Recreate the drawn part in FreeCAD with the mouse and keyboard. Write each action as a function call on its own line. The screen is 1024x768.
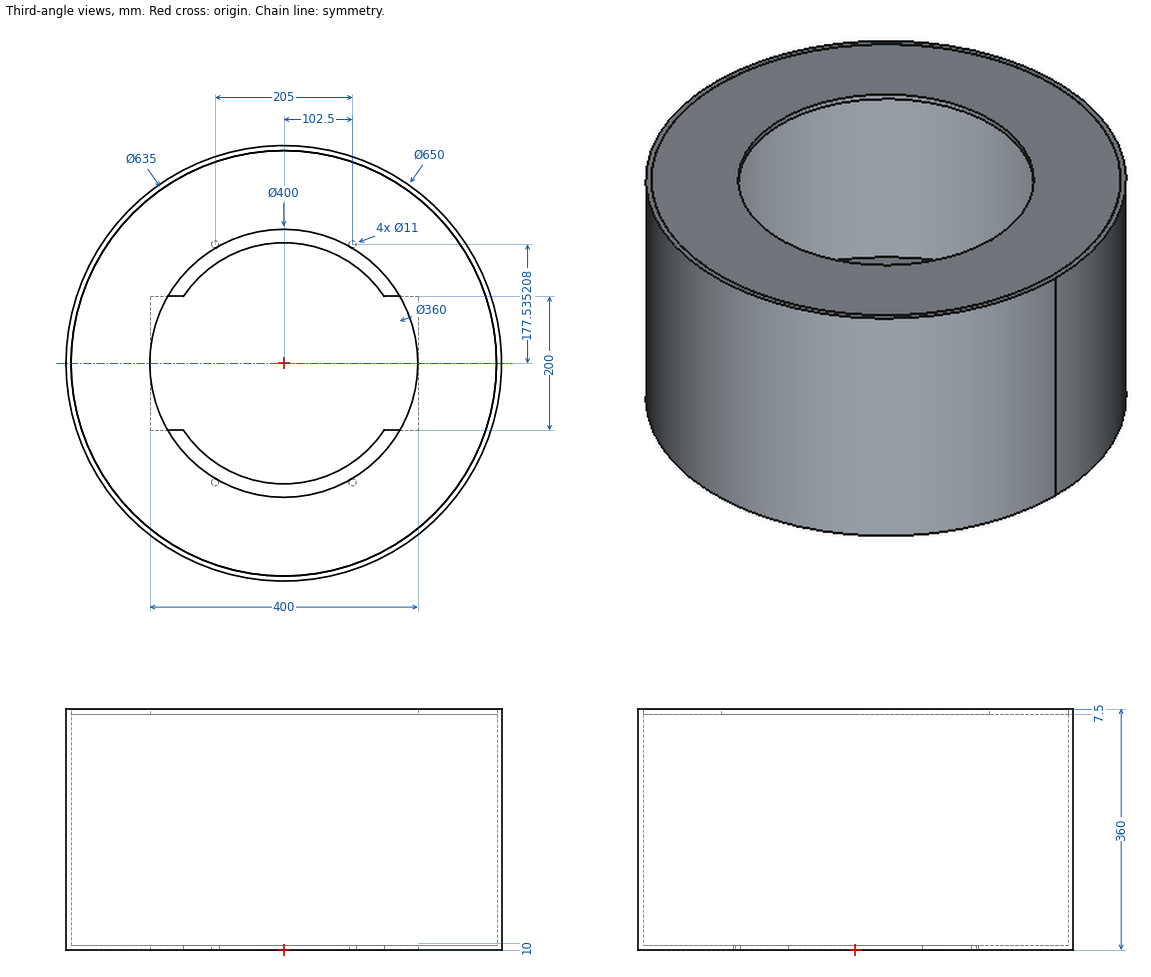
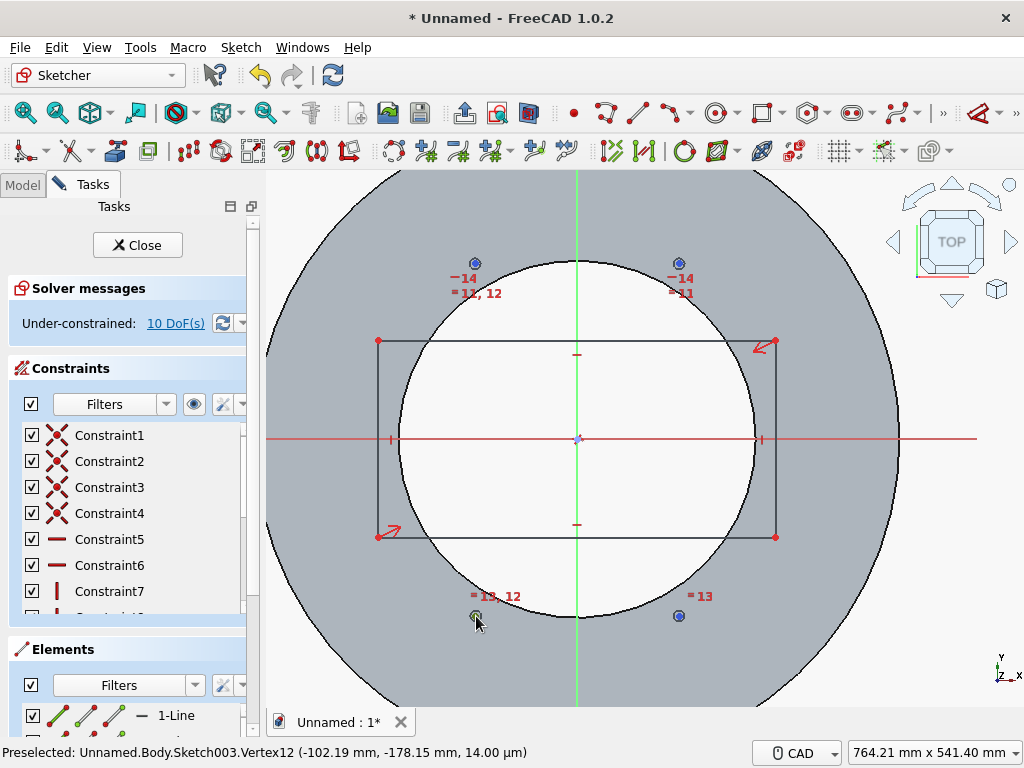
click(679, 616)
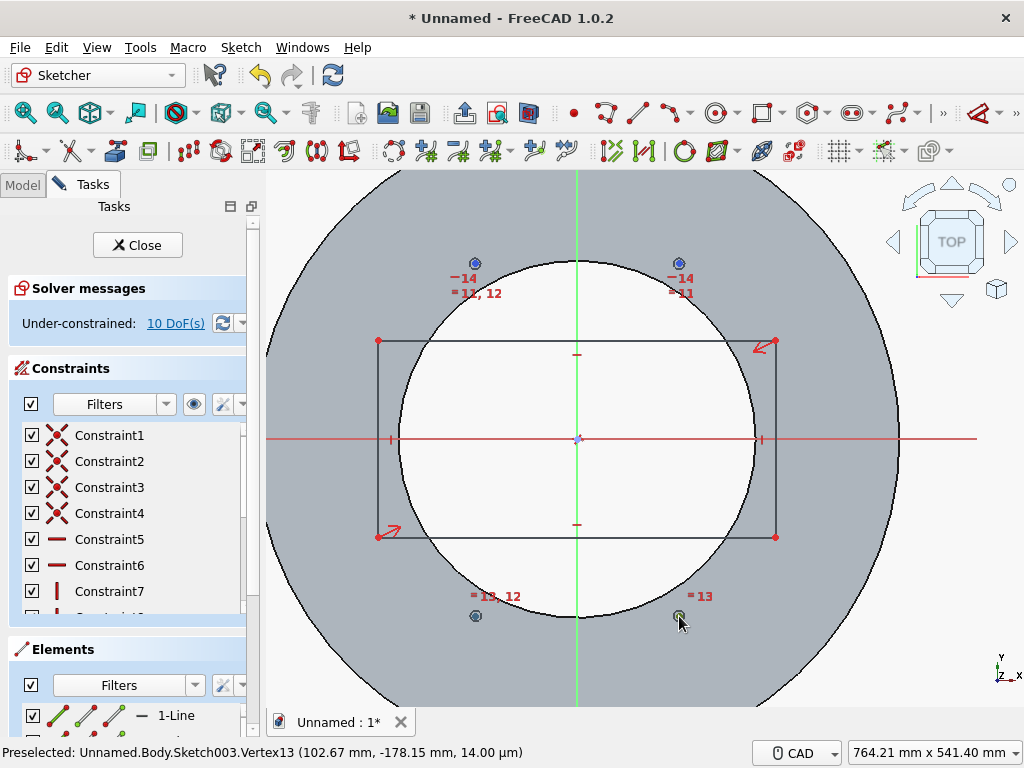
key(h)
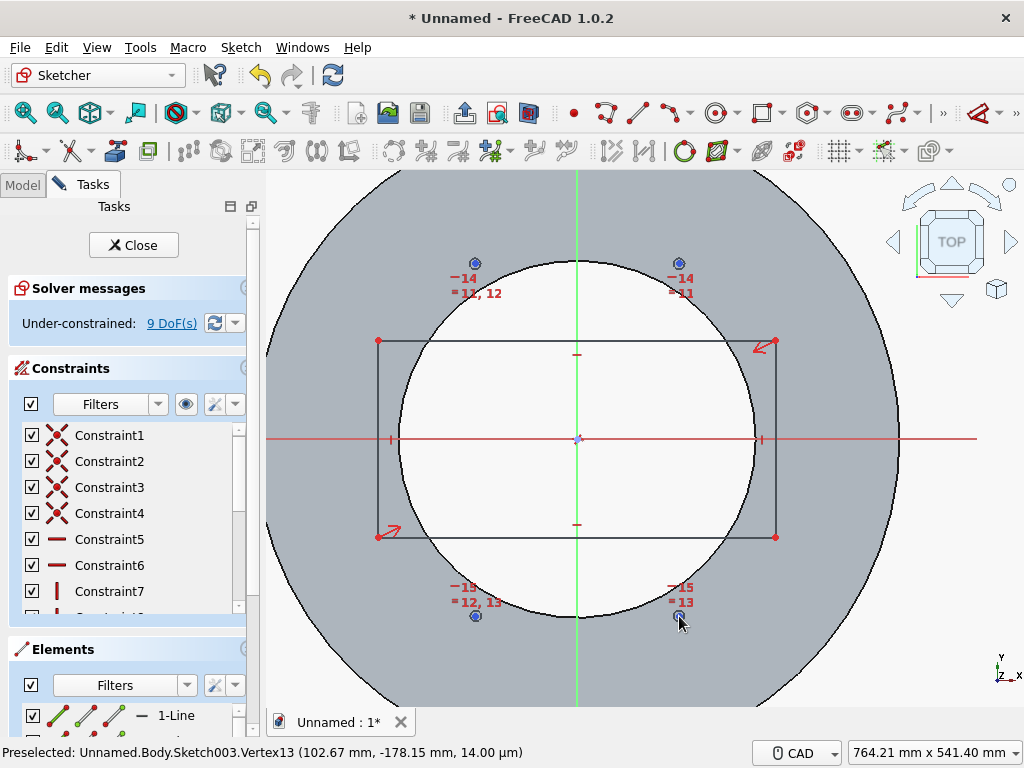
click(475, 264)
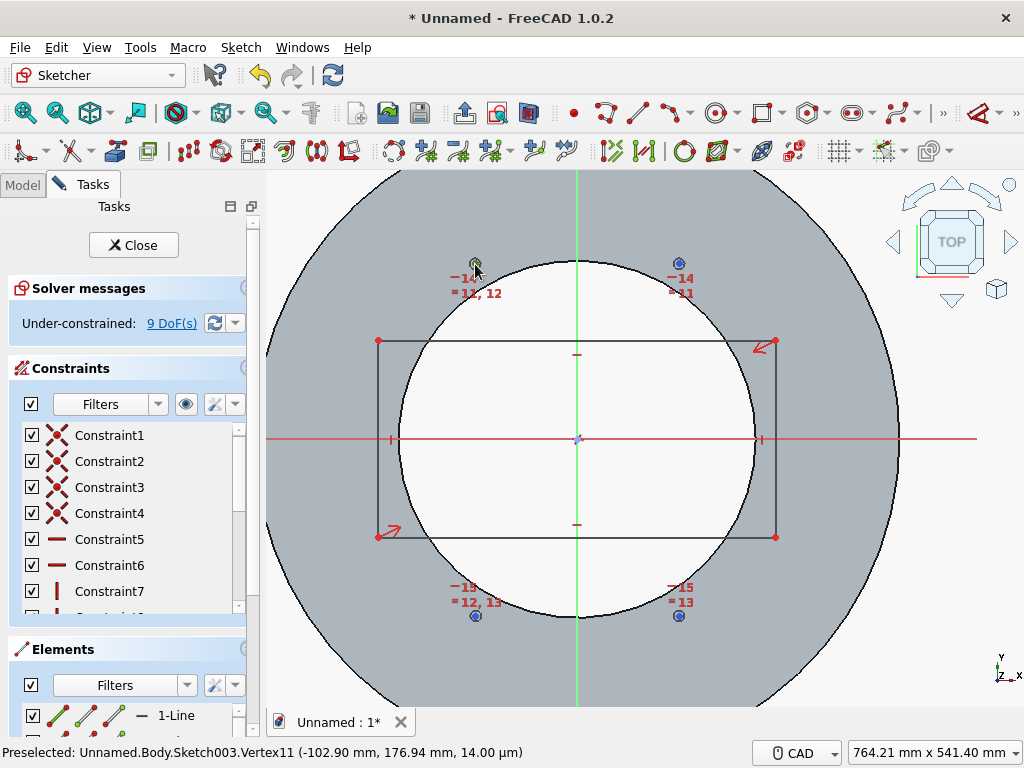
click(476, 616)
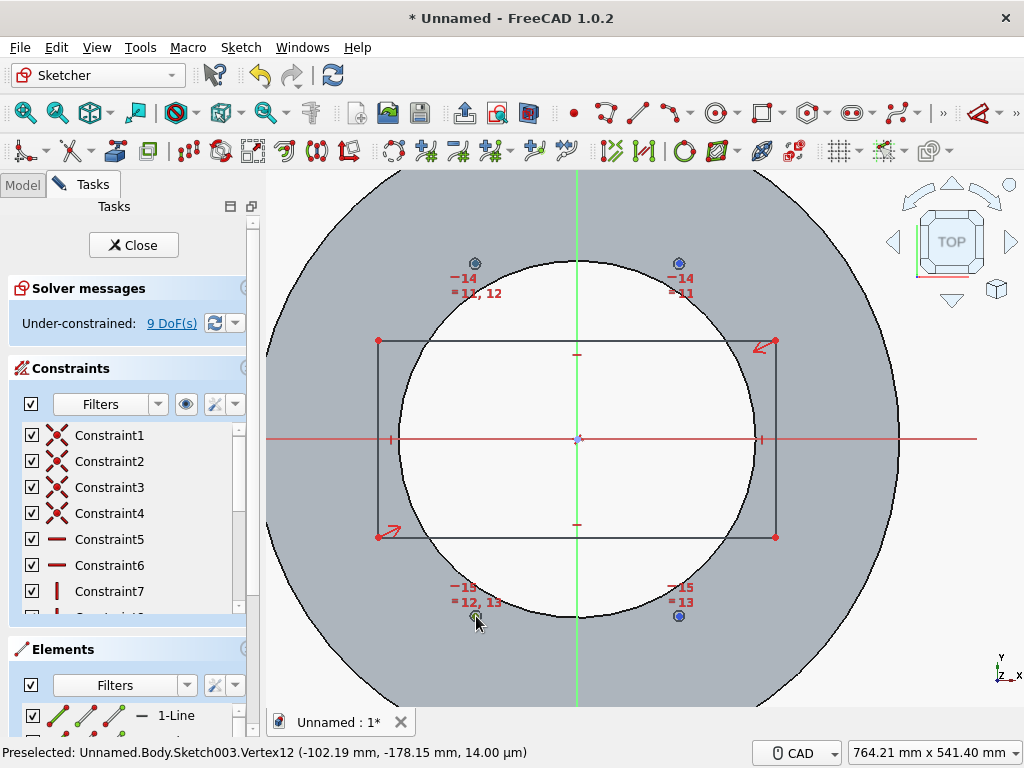
click(334, 439)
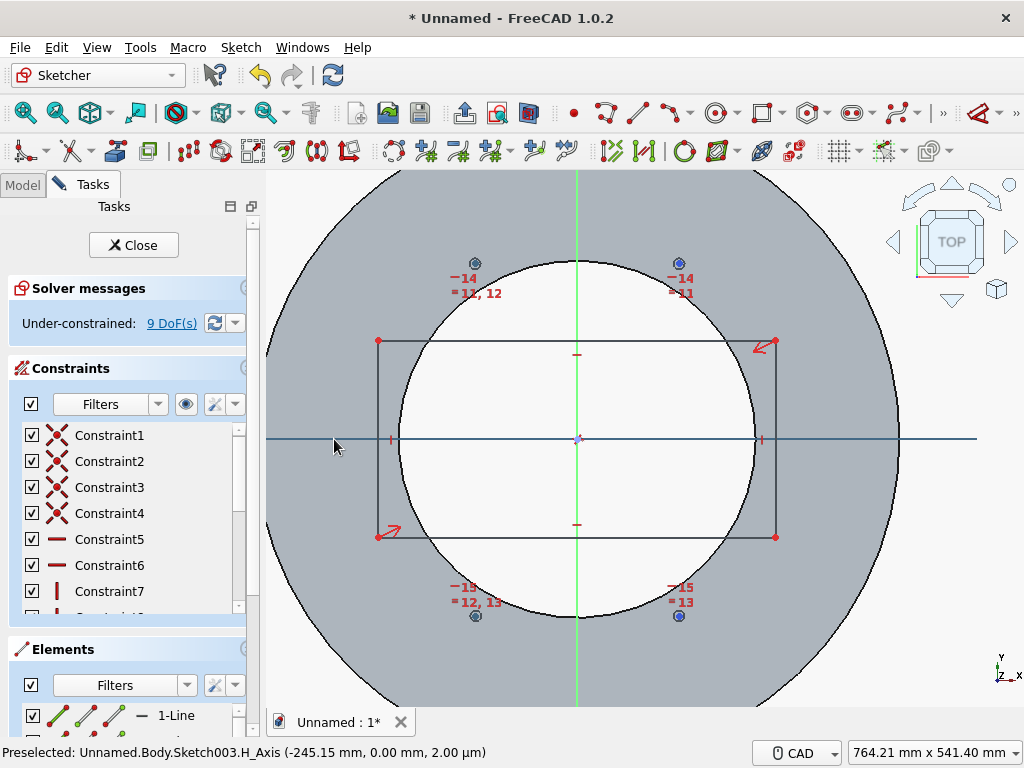
key(s)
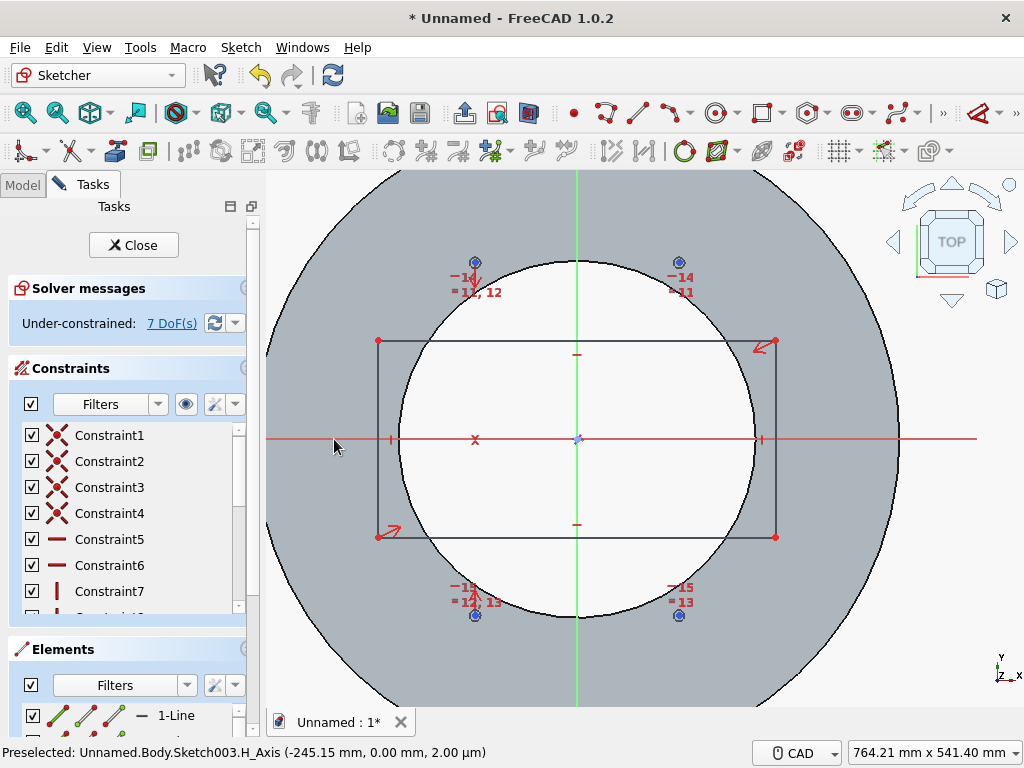
click(978, 114)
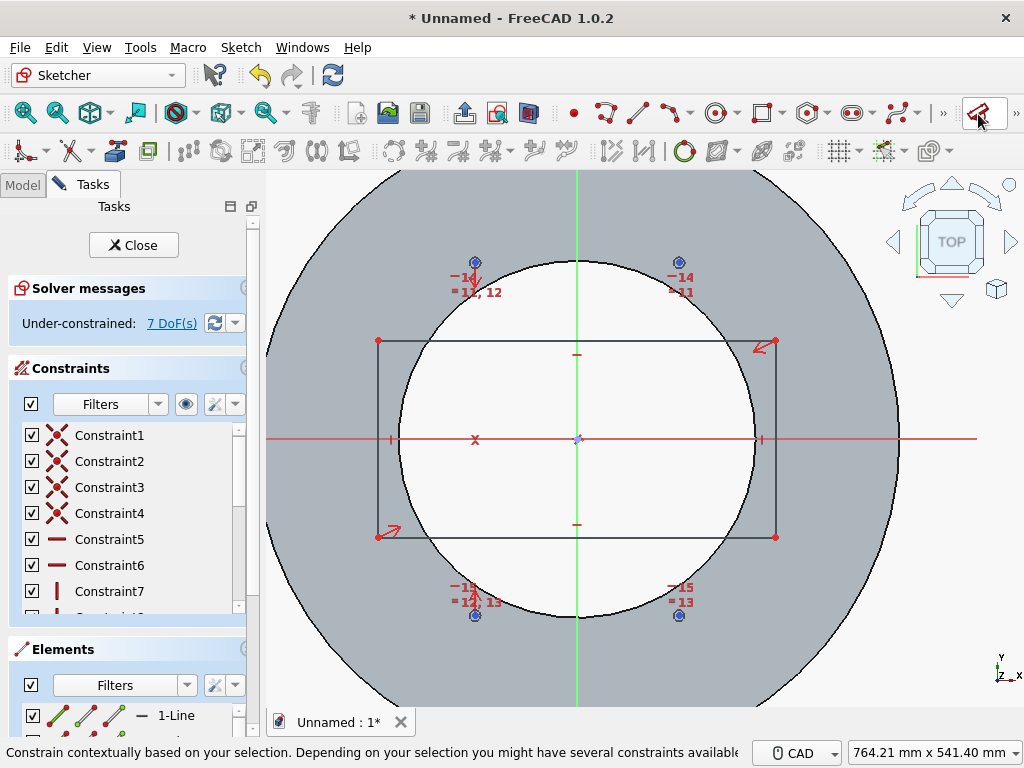
scroll(679, 257, up, 7)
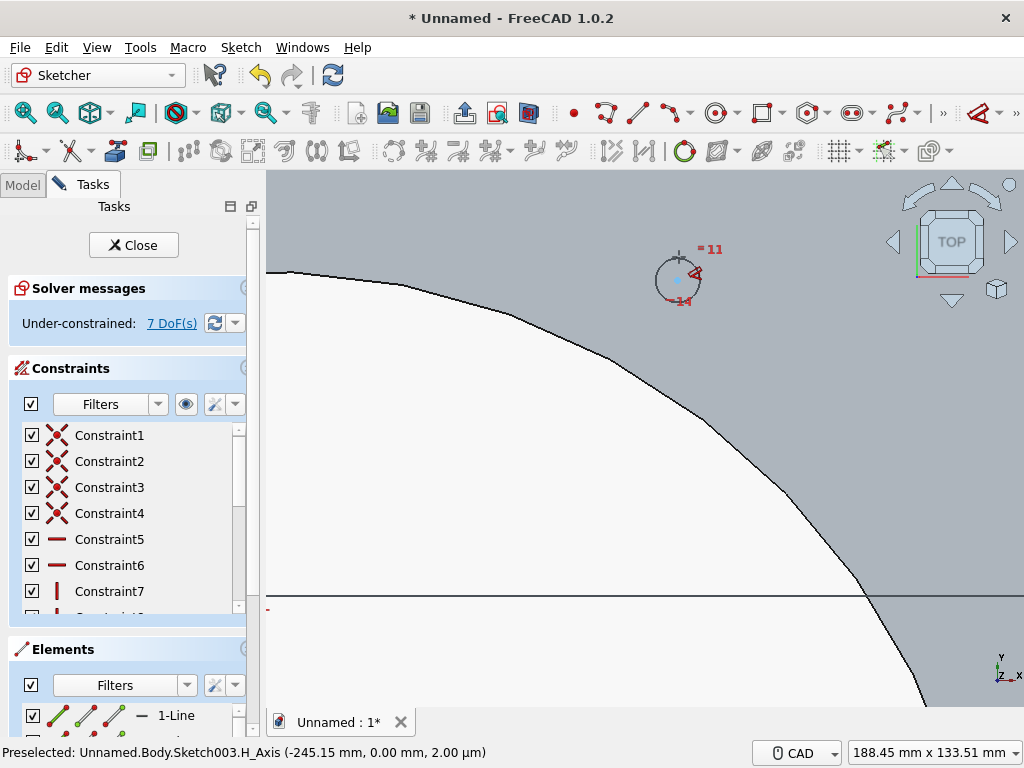
click(678, 258)
click(678, 226)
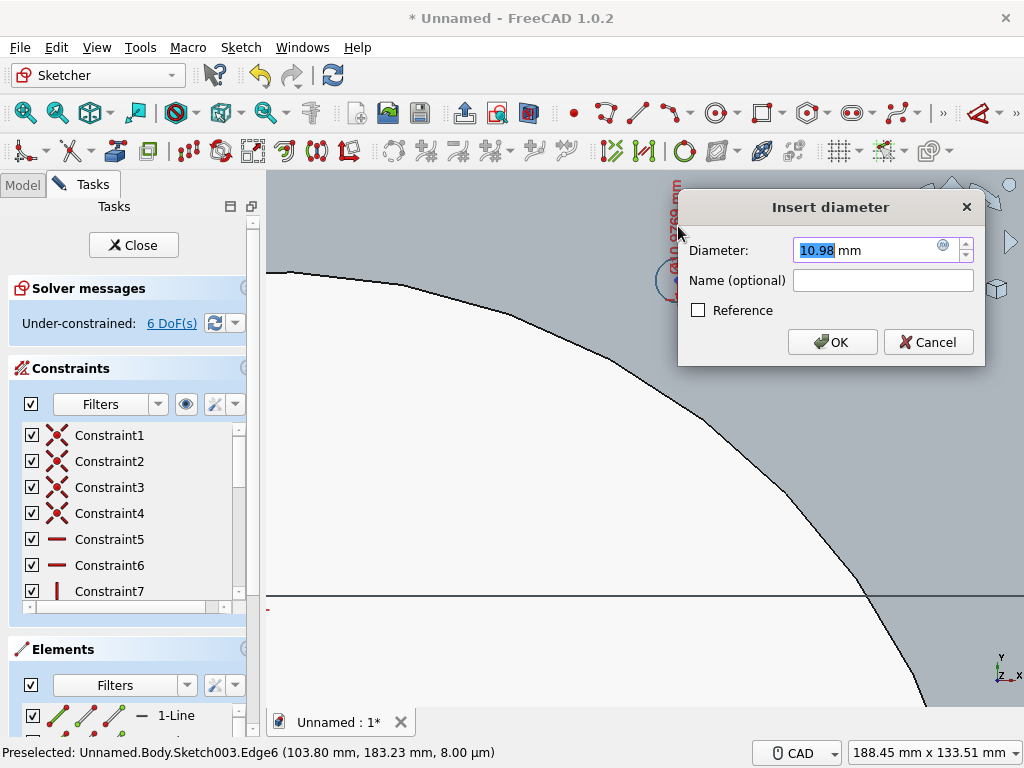
text(11)
key(Return)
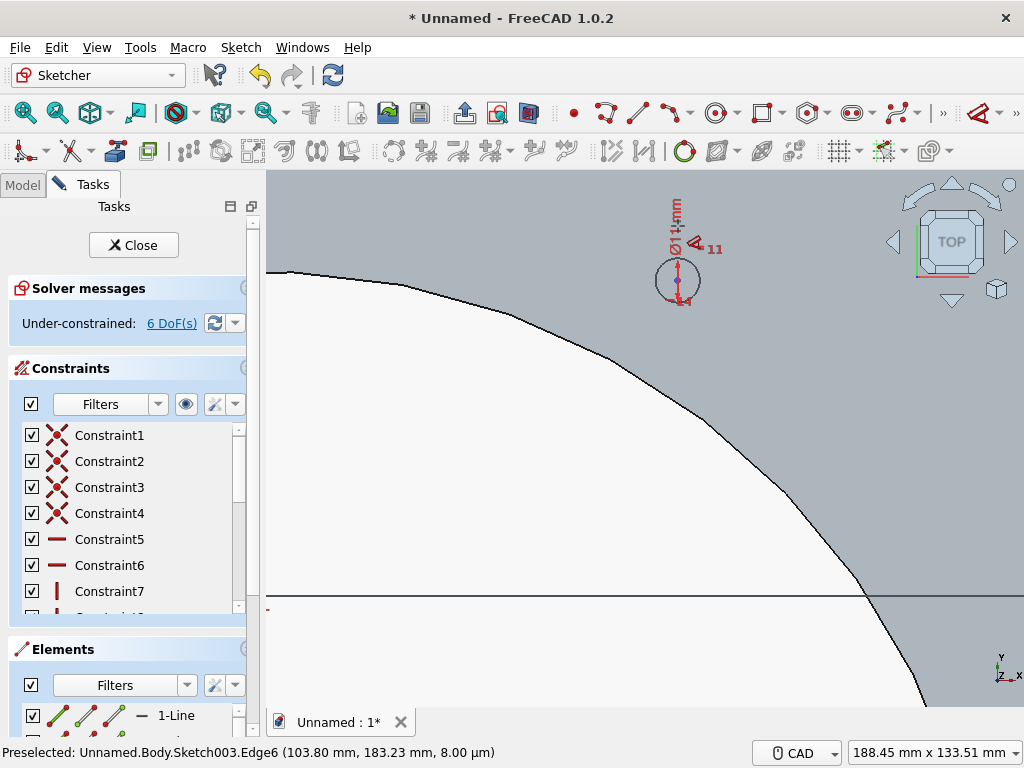
scroll(679, 256, down, 7)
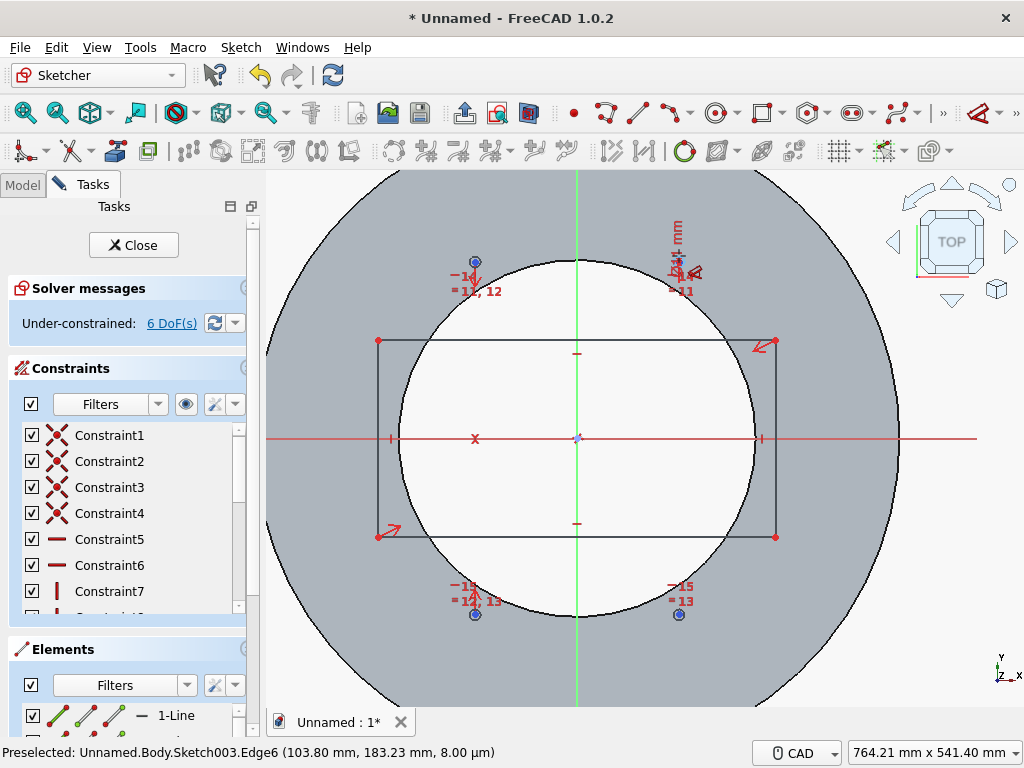
click(498, 537)
click(486, 571)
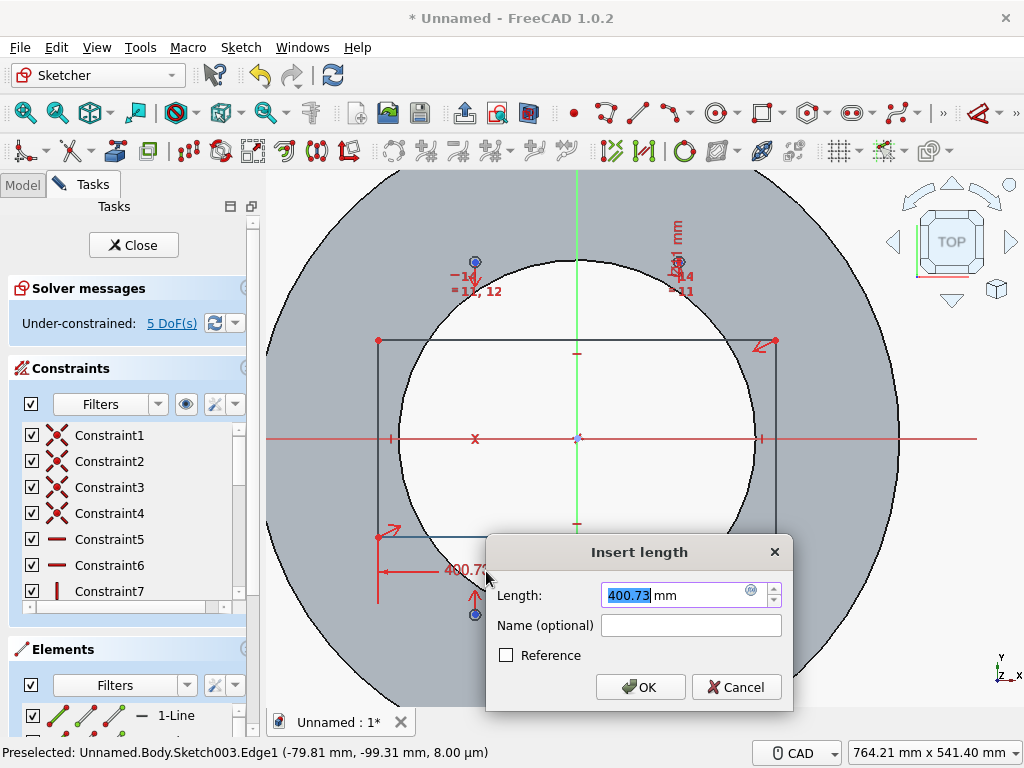
text(400)
key(Return)